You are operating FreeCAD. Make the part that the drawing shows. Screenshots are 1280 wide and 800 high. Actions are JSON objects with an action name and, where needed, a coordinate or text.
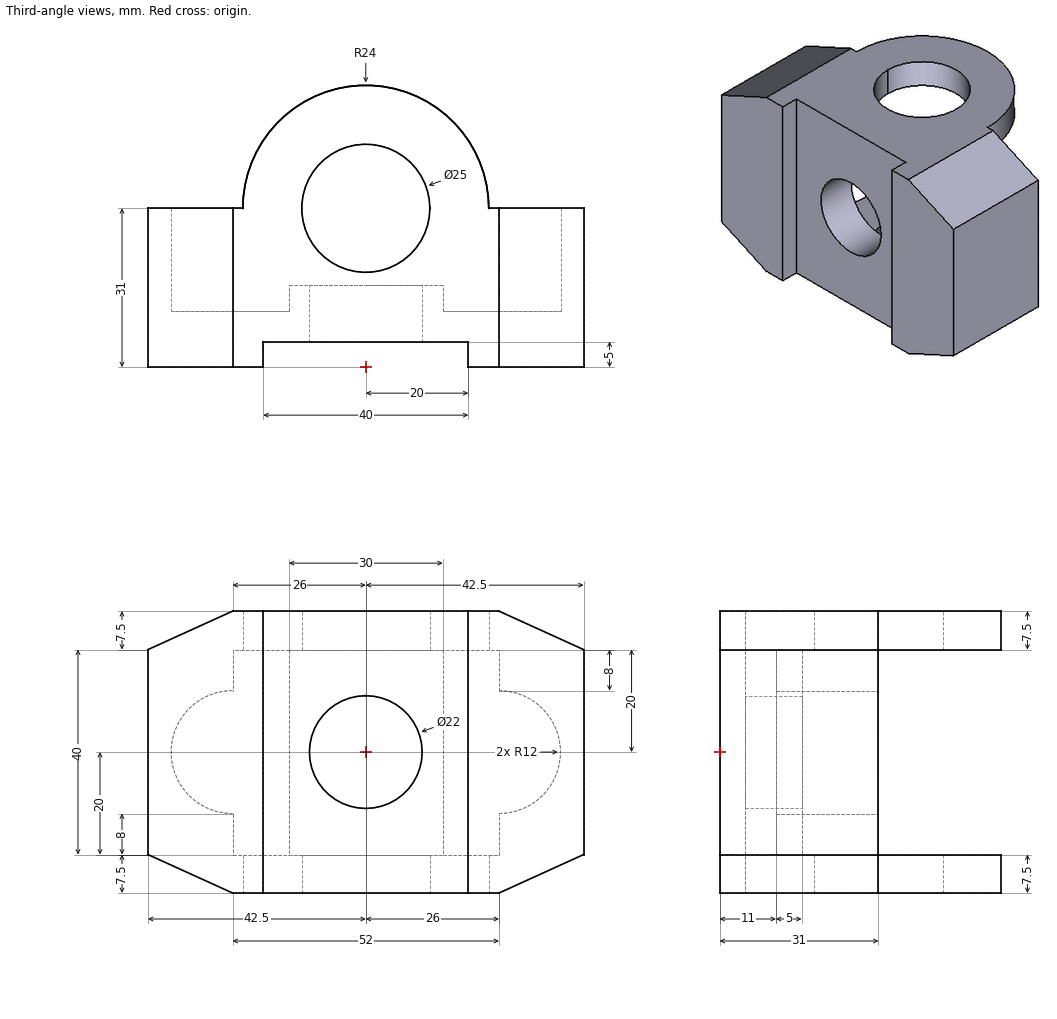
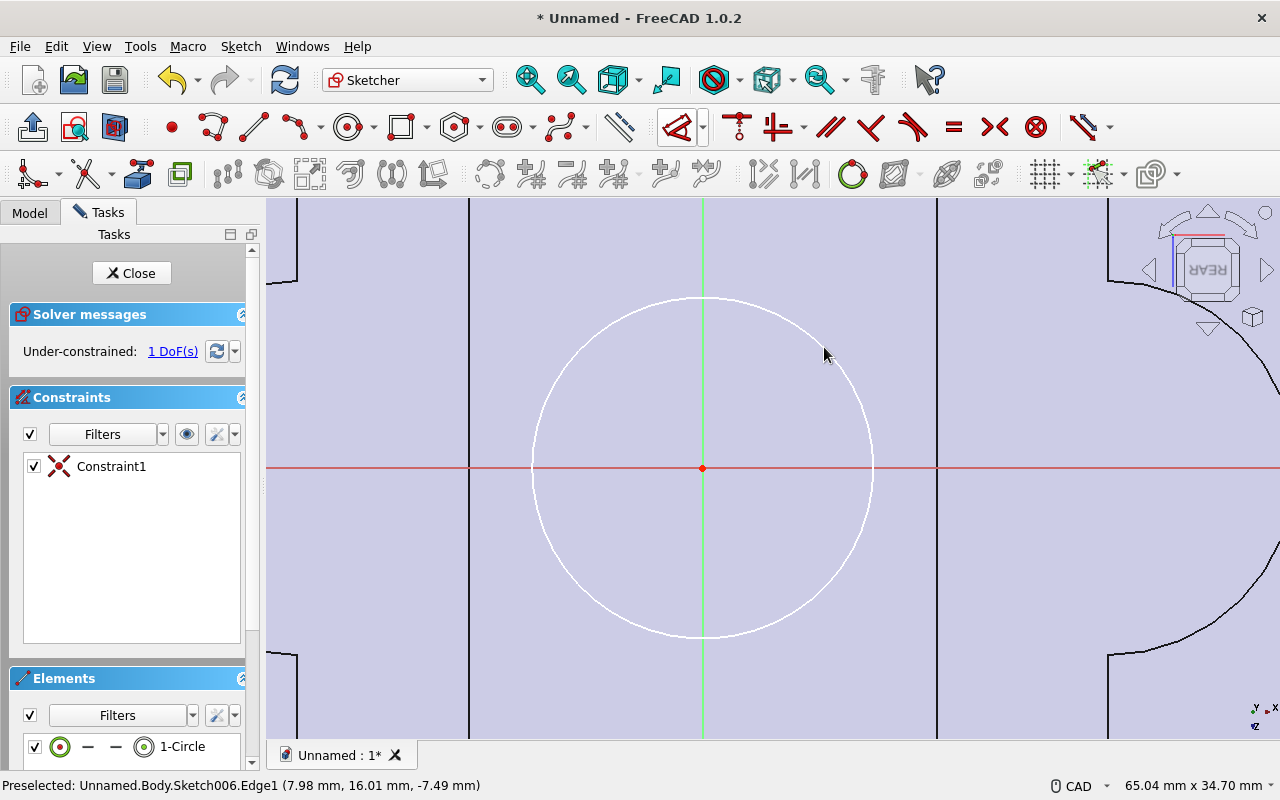
{"action": "left_click", "coordinate": [823, 347]}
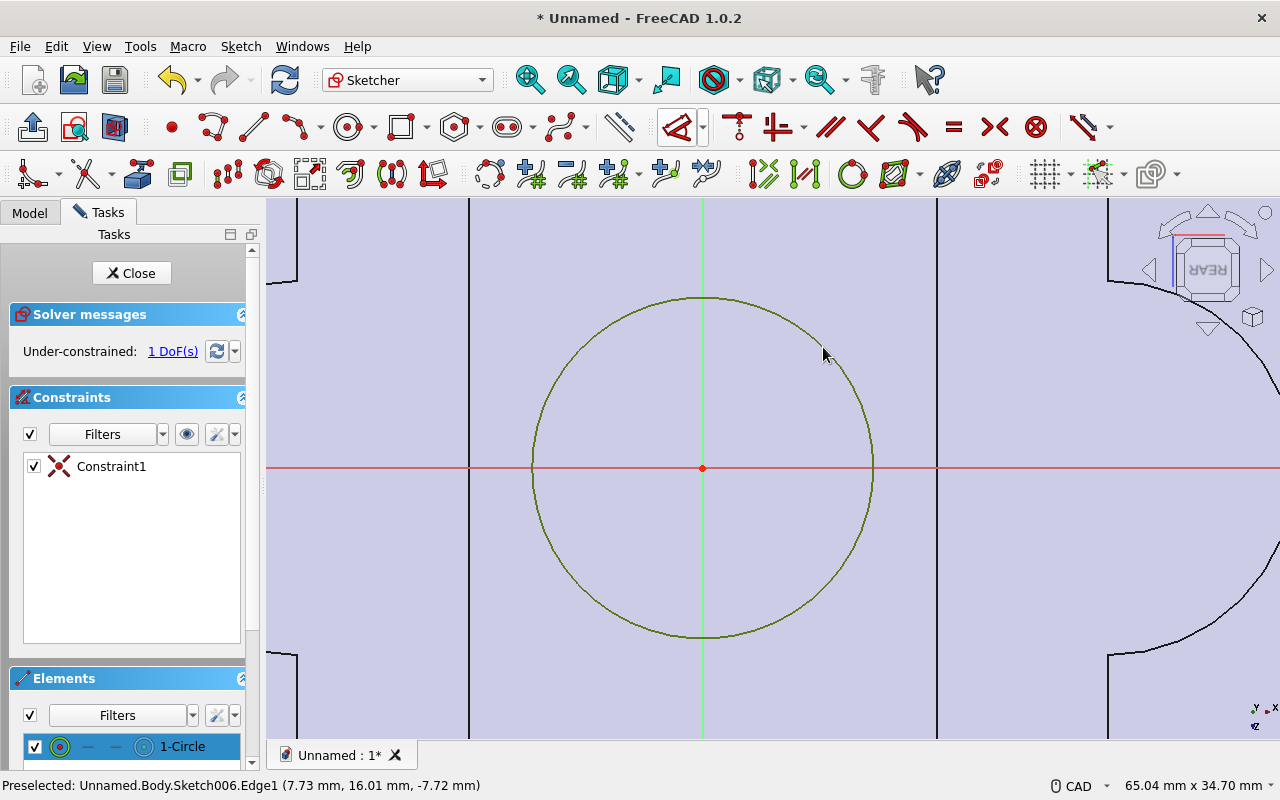
{"action": "key", "text": "k o"}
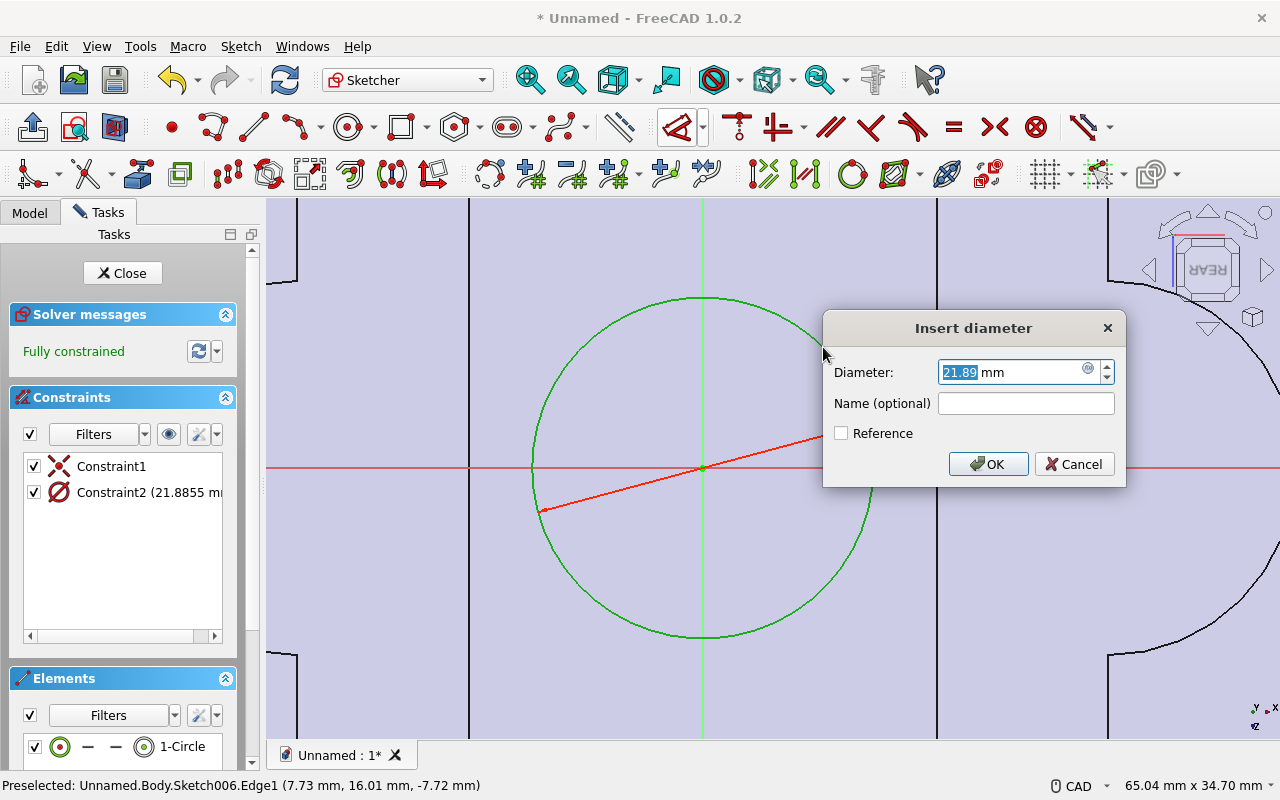
{"action": "type", "text": "22"}
{"action": "key", "text": "Return"}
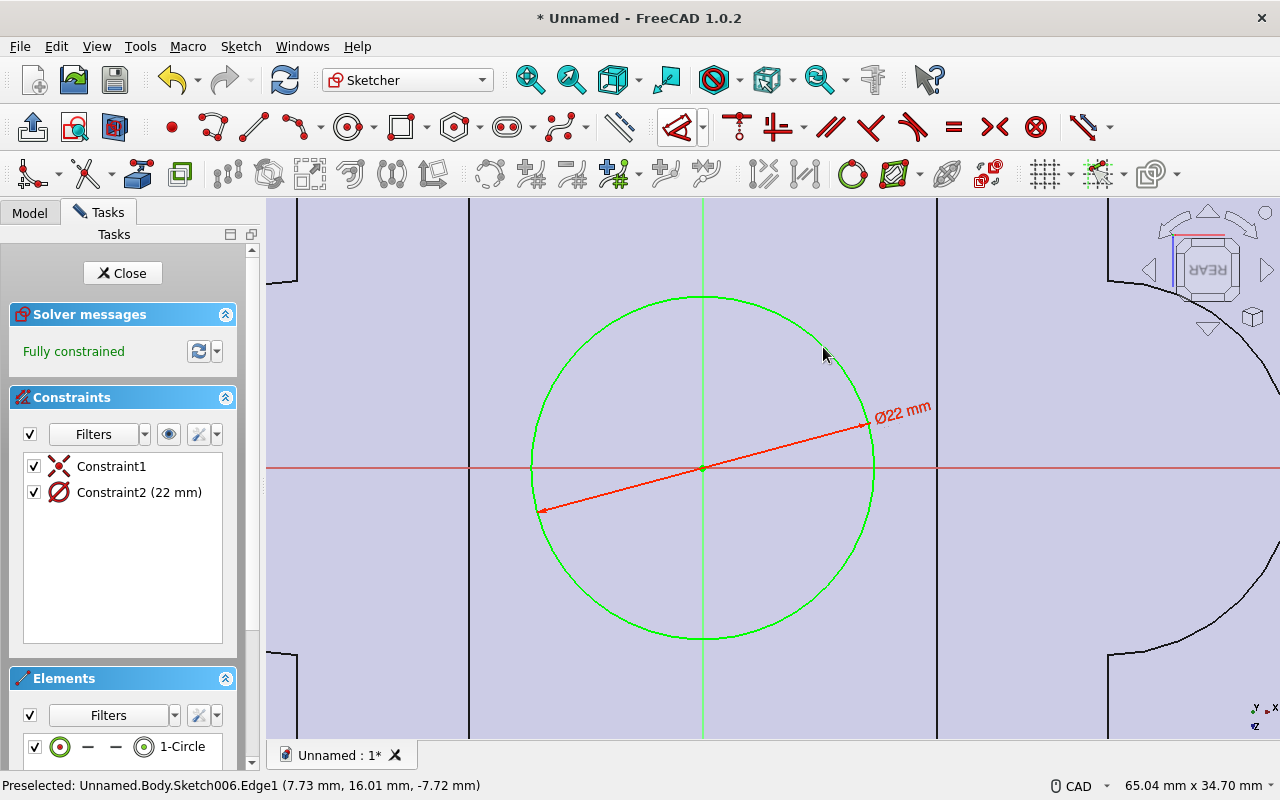
{"action": "left_click", "coordinate": [123, 273]}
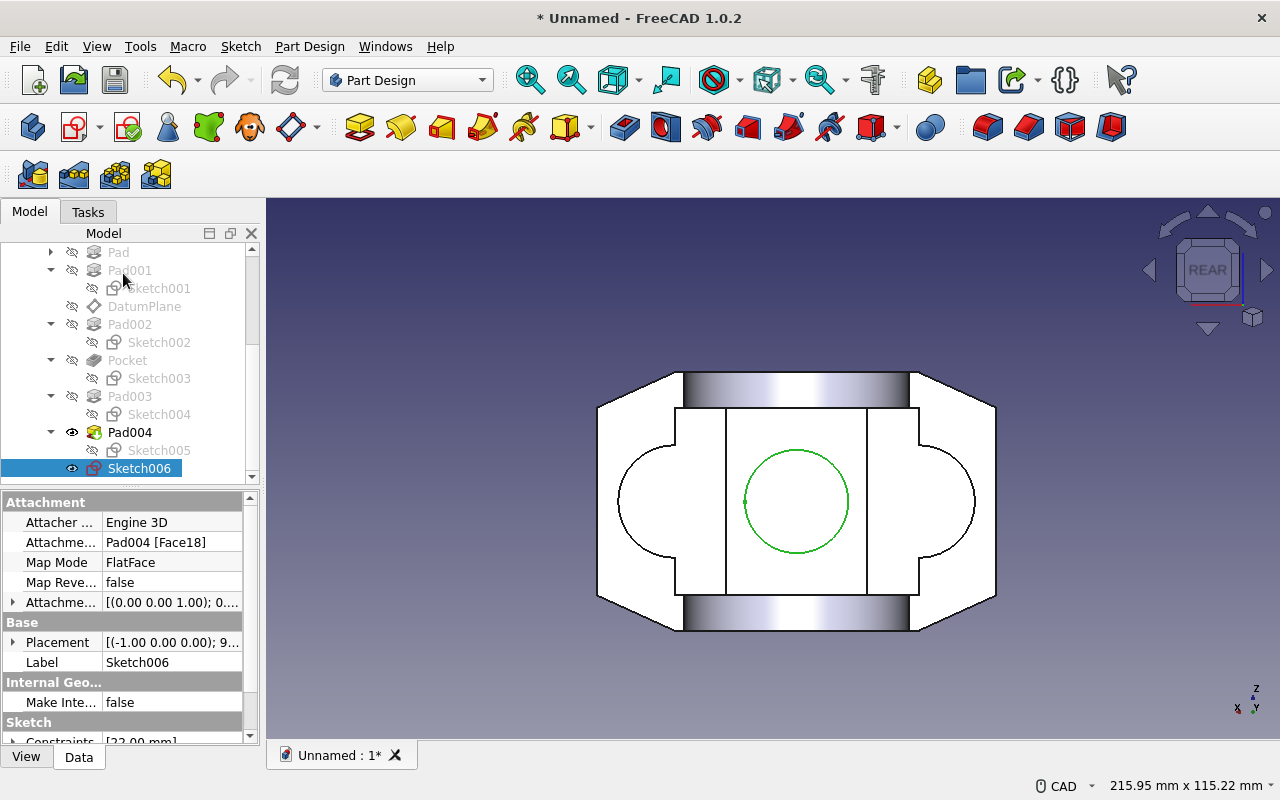
{"action": "left_click", "coordinate": [625, 128]}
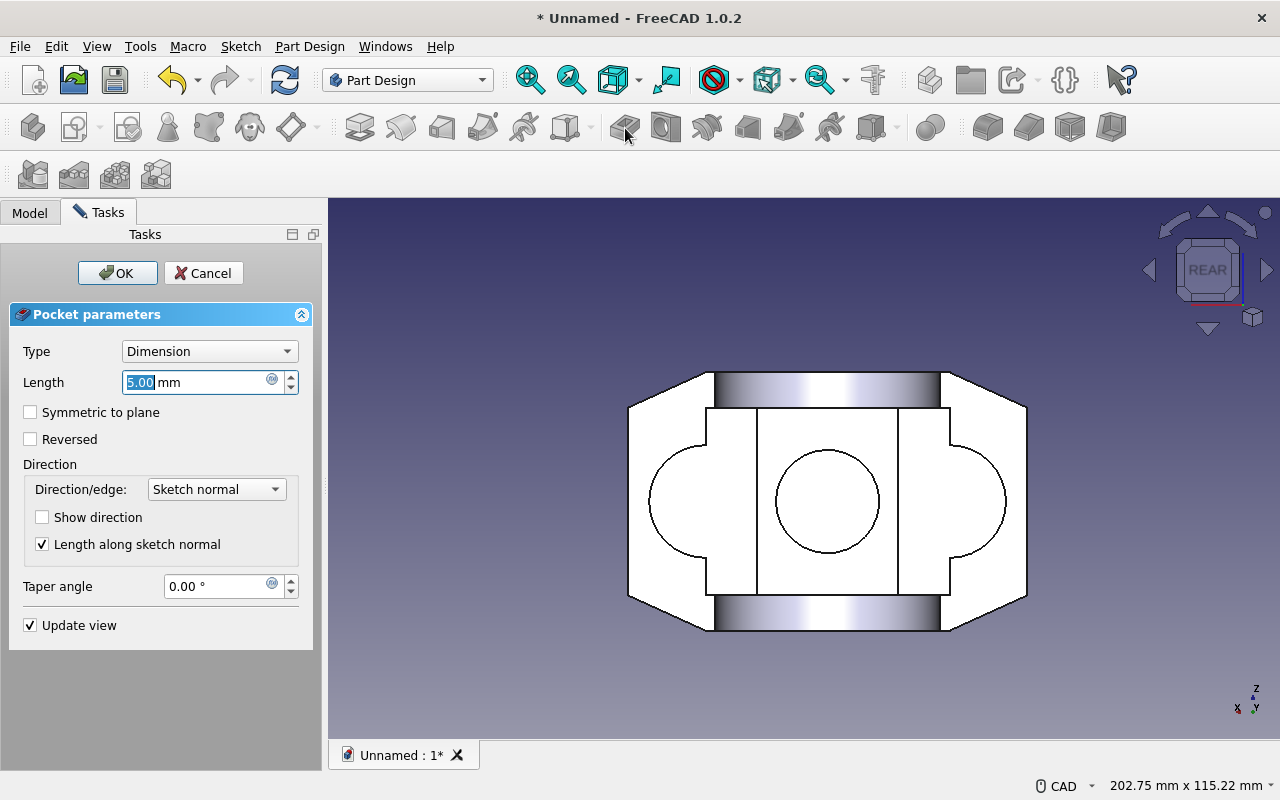
{"action": "left_click", "coordinate": [210, 352]}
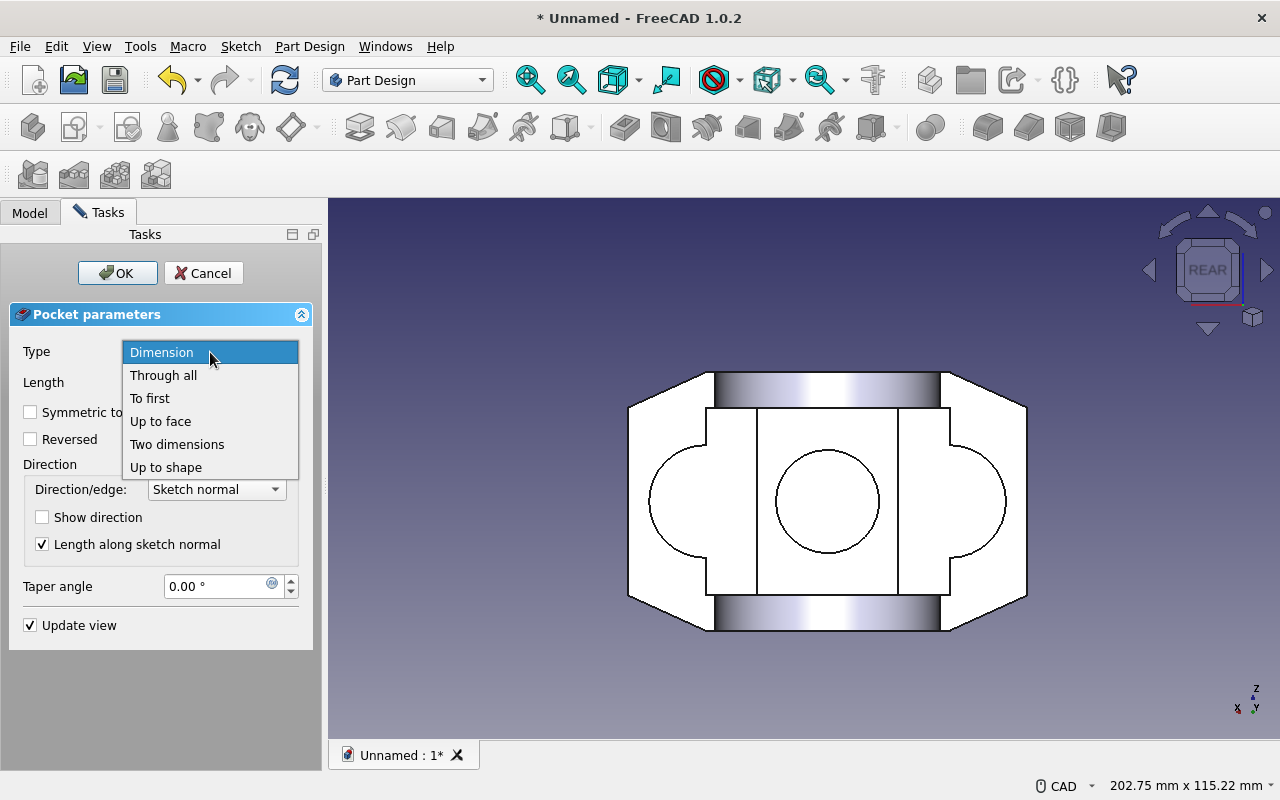
{"action": "left_click", "coordinate": [208, 398]}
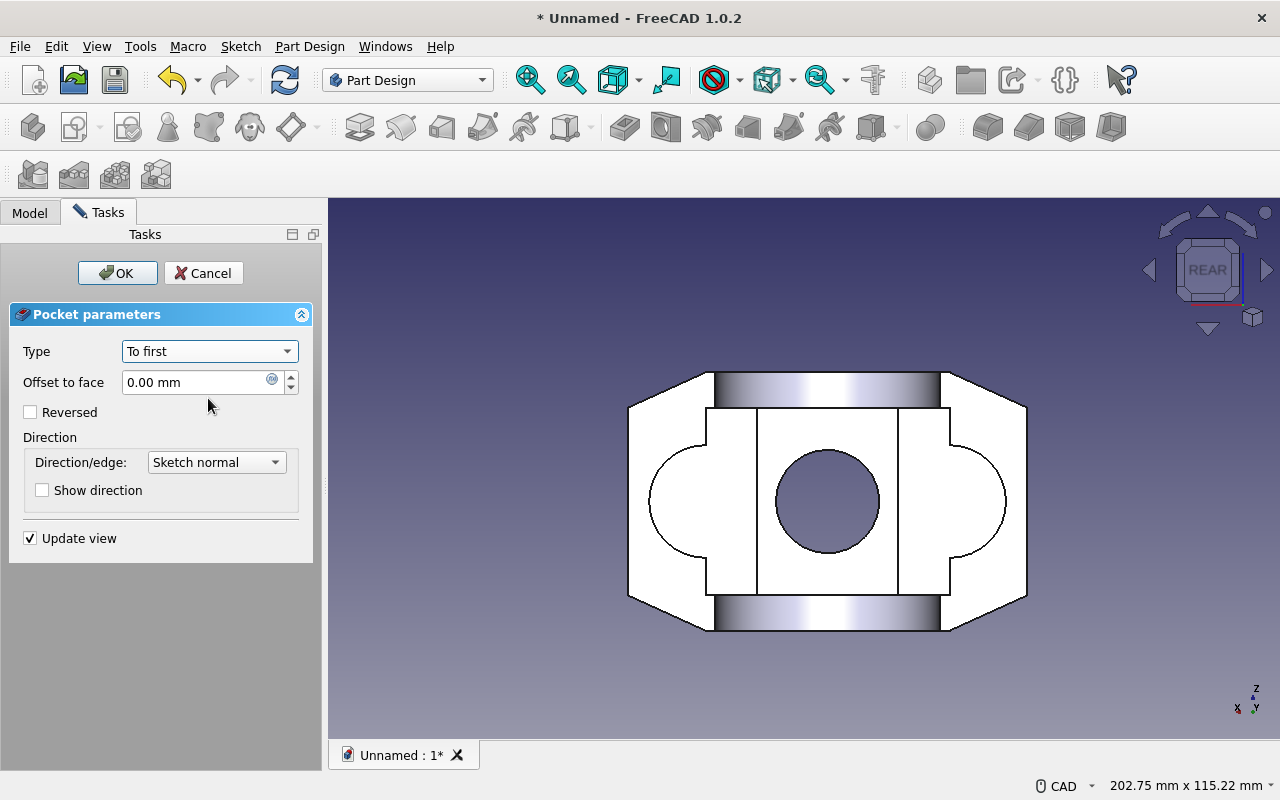
{"action": "left_click", "coordinate": [118, 273]}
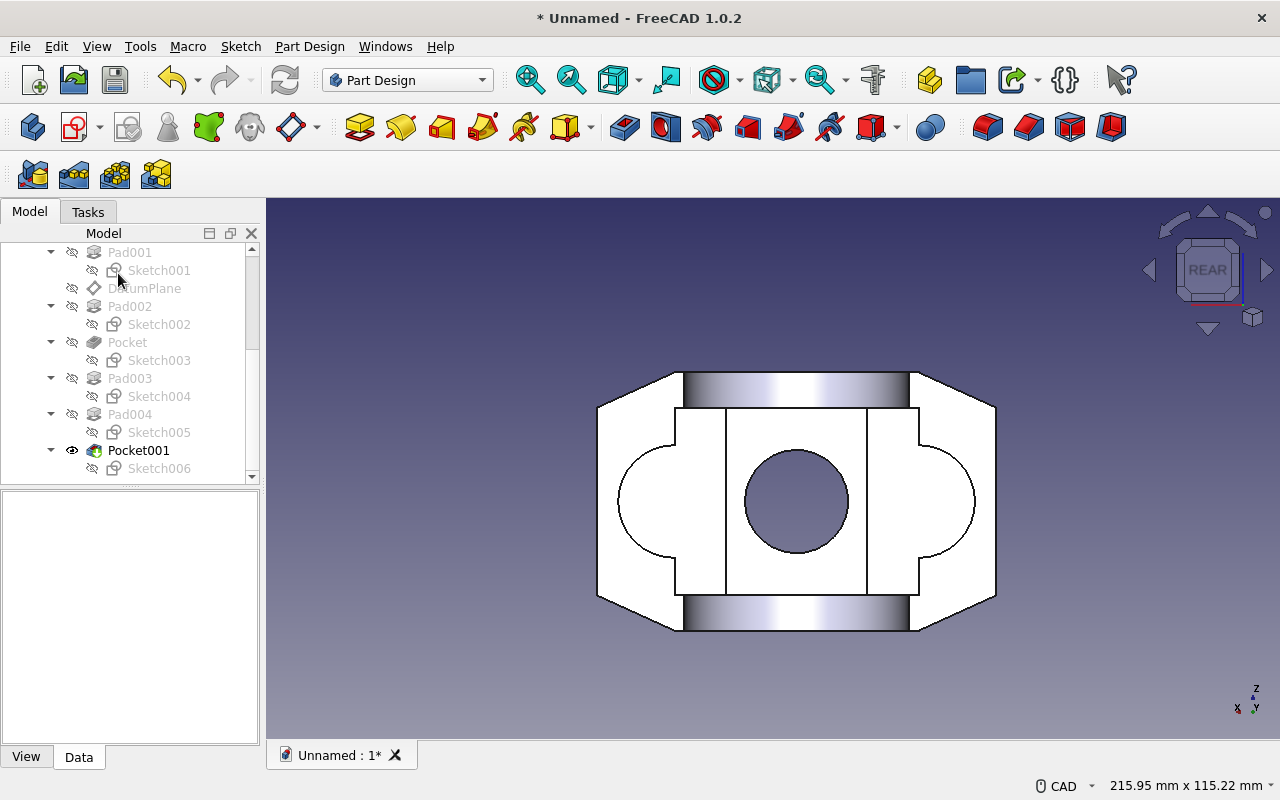
{"action": "key", "text": "0"}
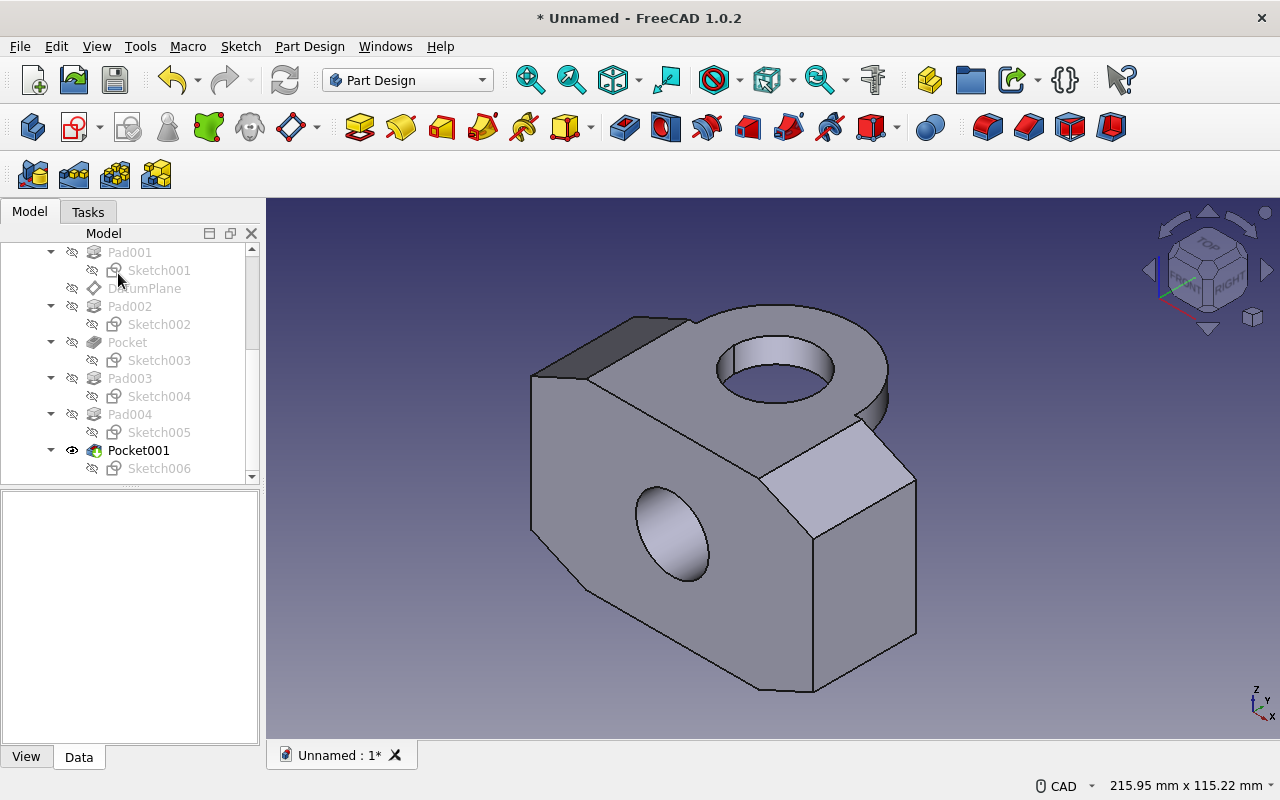
{"action": "left_click", "coordinate": [761, 434]}